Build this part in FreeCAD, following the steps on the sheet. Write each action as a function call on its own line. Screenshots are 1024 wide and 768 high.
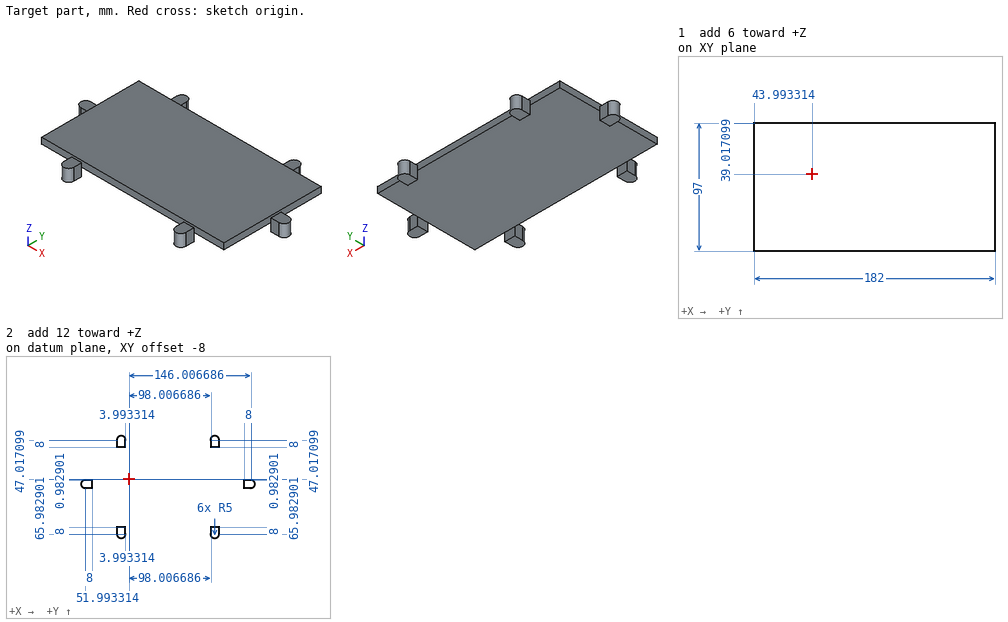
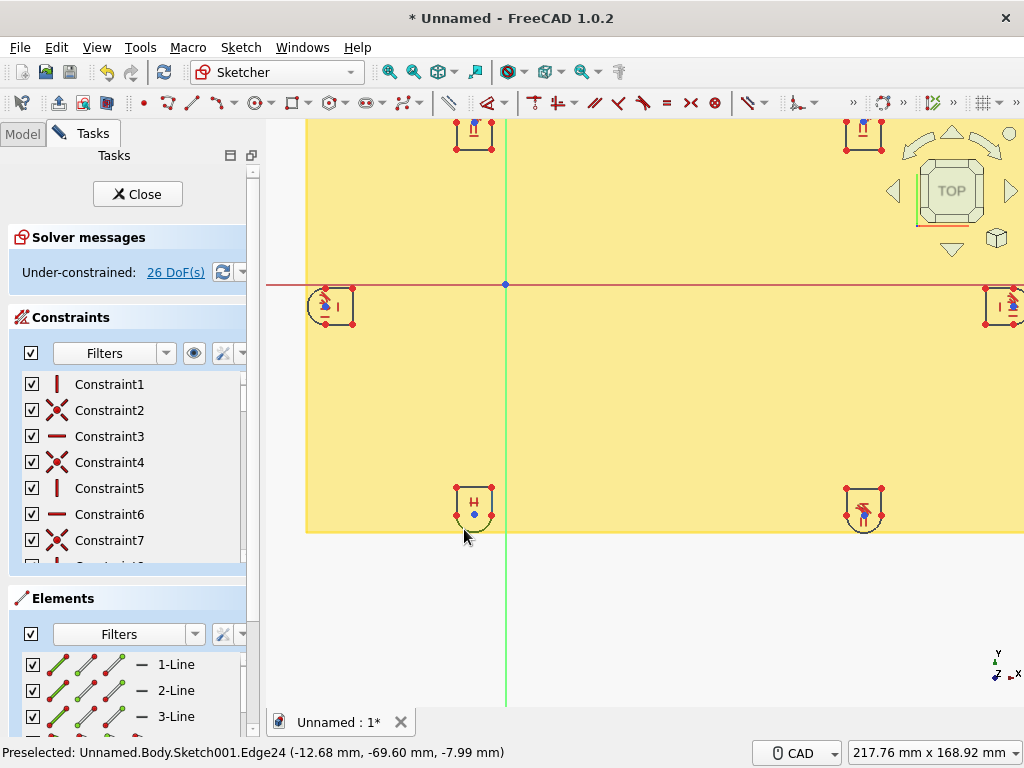
click(644, 104)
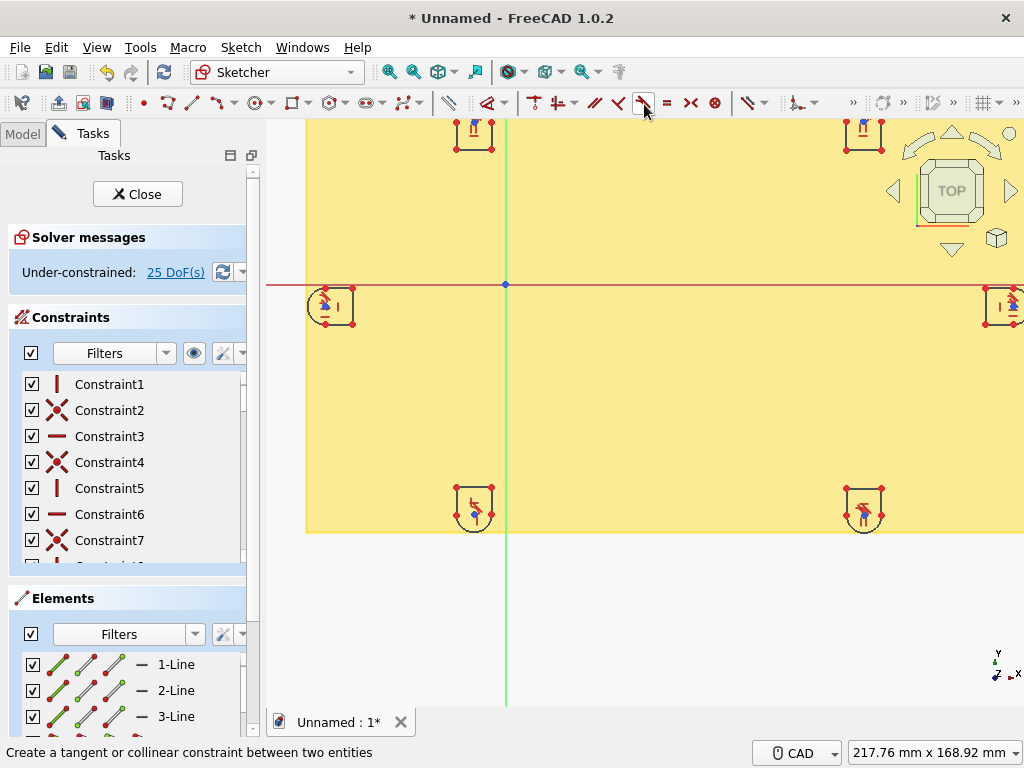
scroll(457, 498, up, 2)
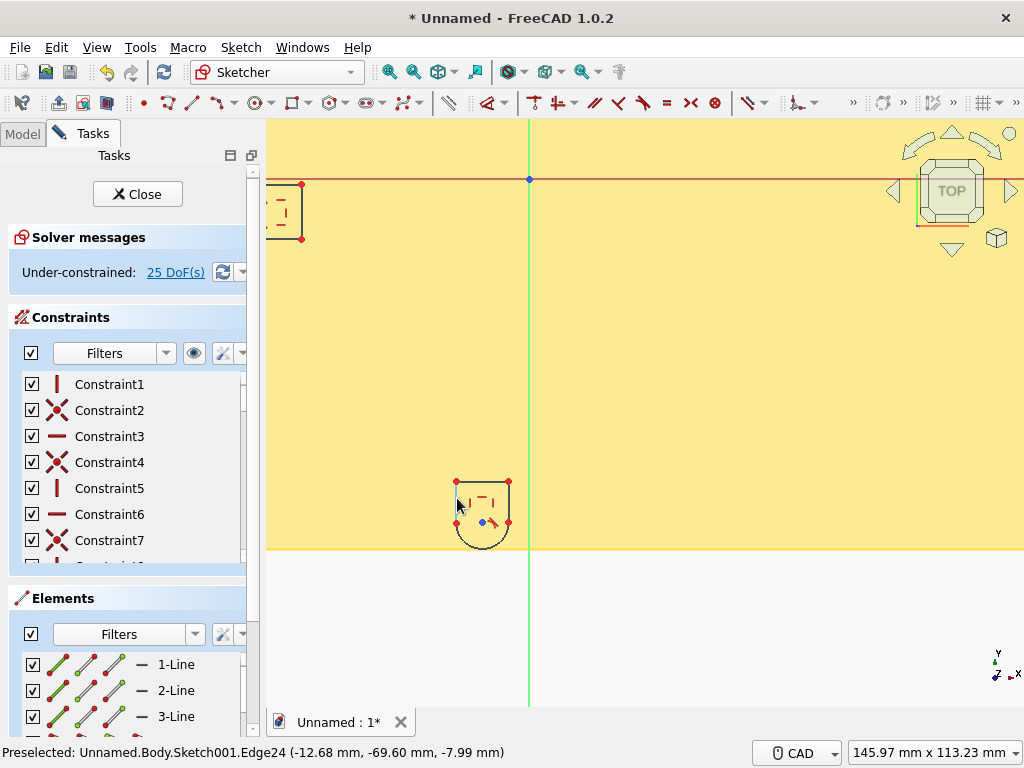
click(456, 498)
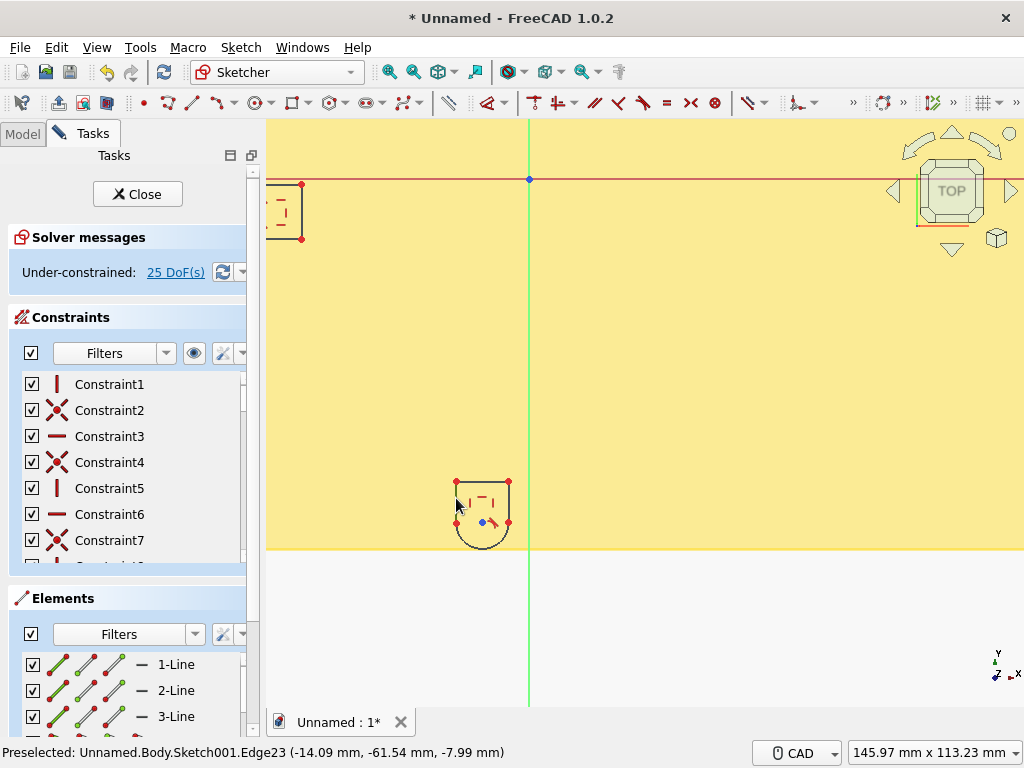
click(467, 544)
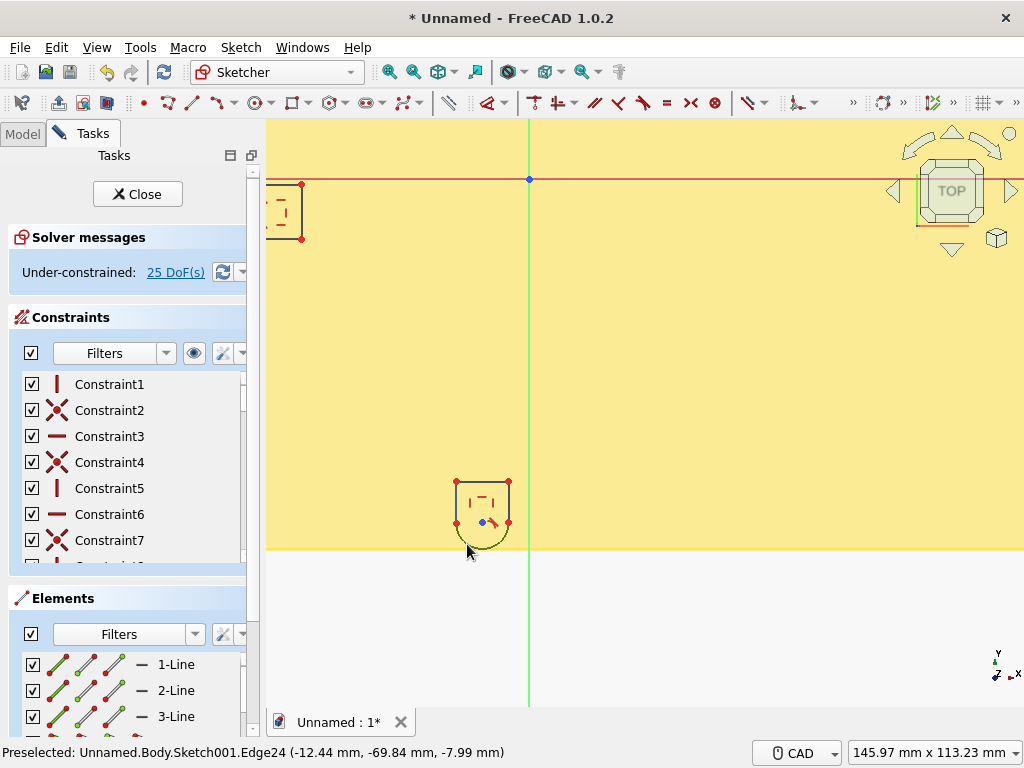
click(644, 104)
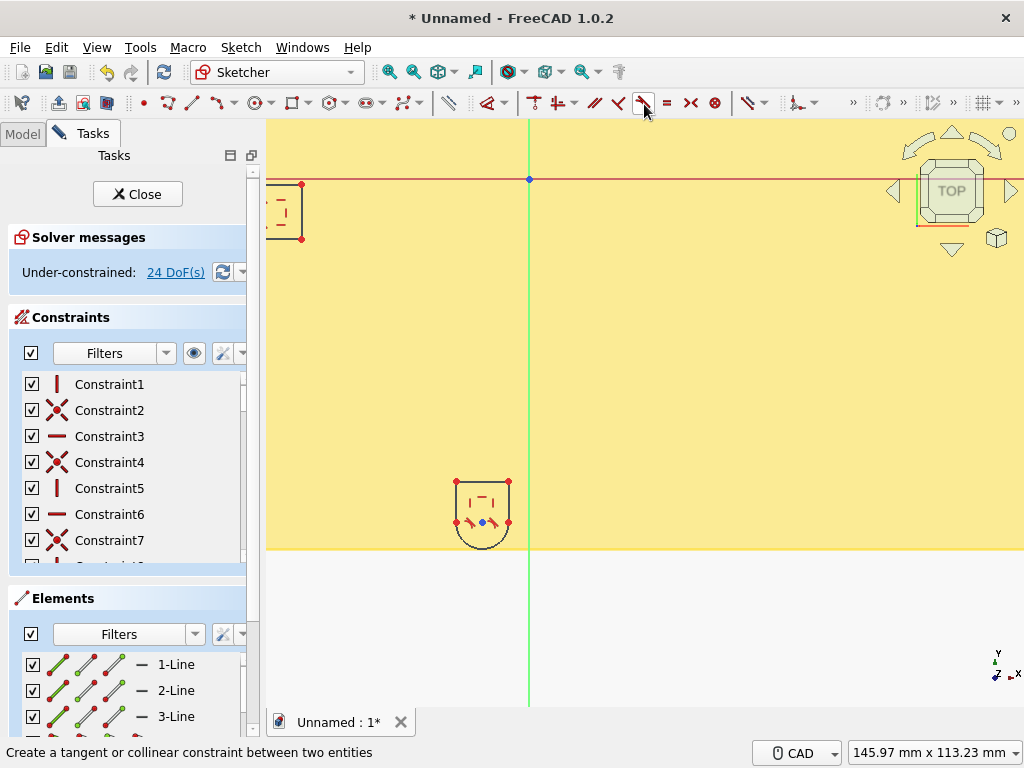
scroll(462, 520, down, 5)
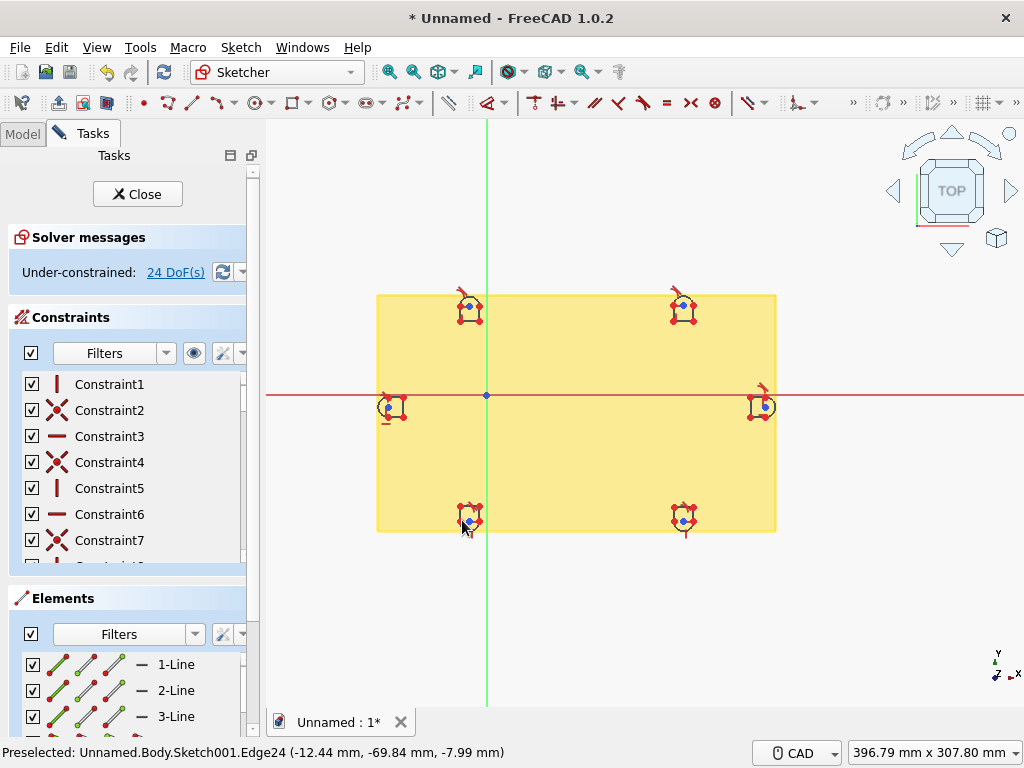
scroll(678, 530, up, 3)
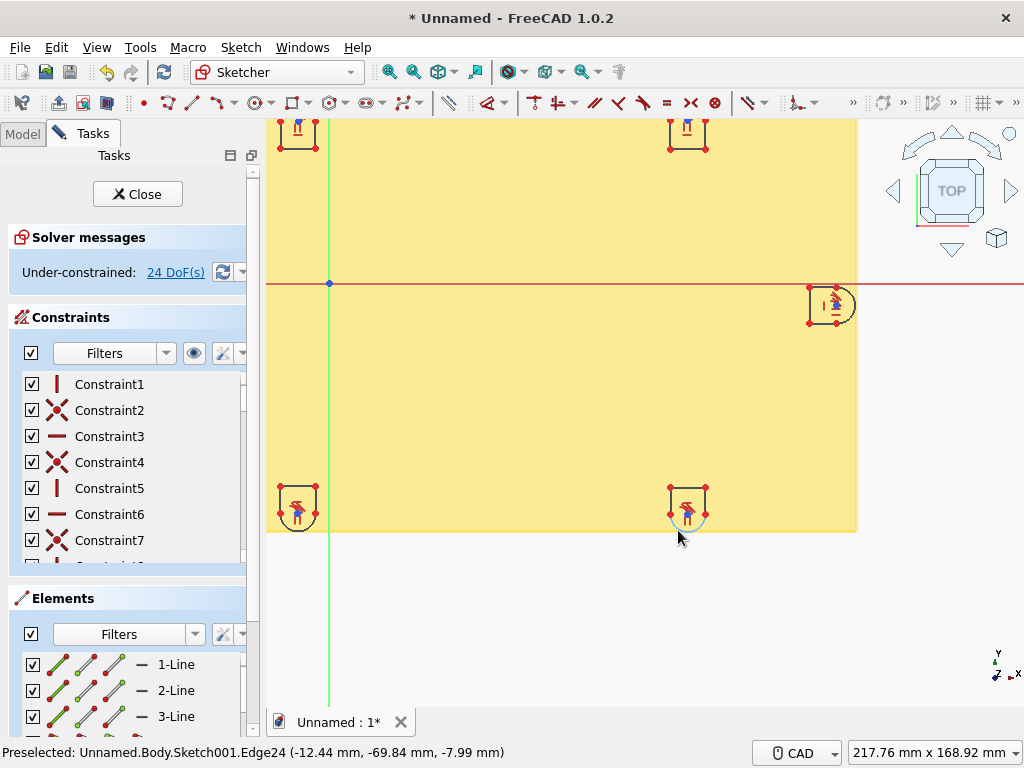
click(678, 529)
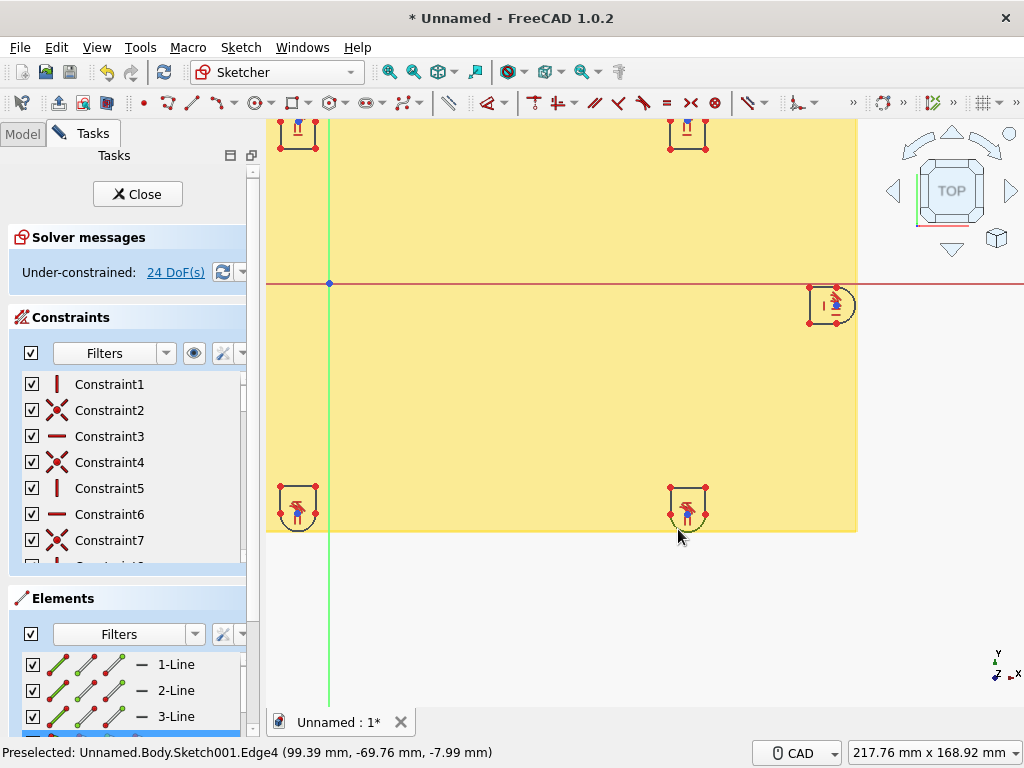
click(852, 316)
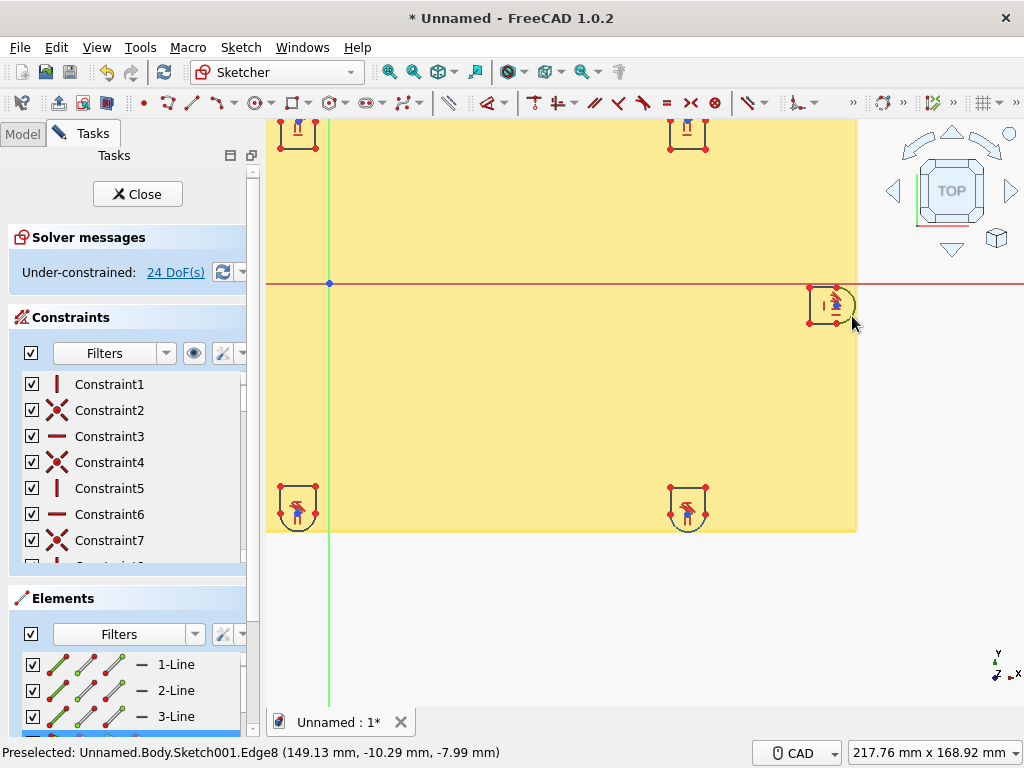
scroll(678, 530, down, 3)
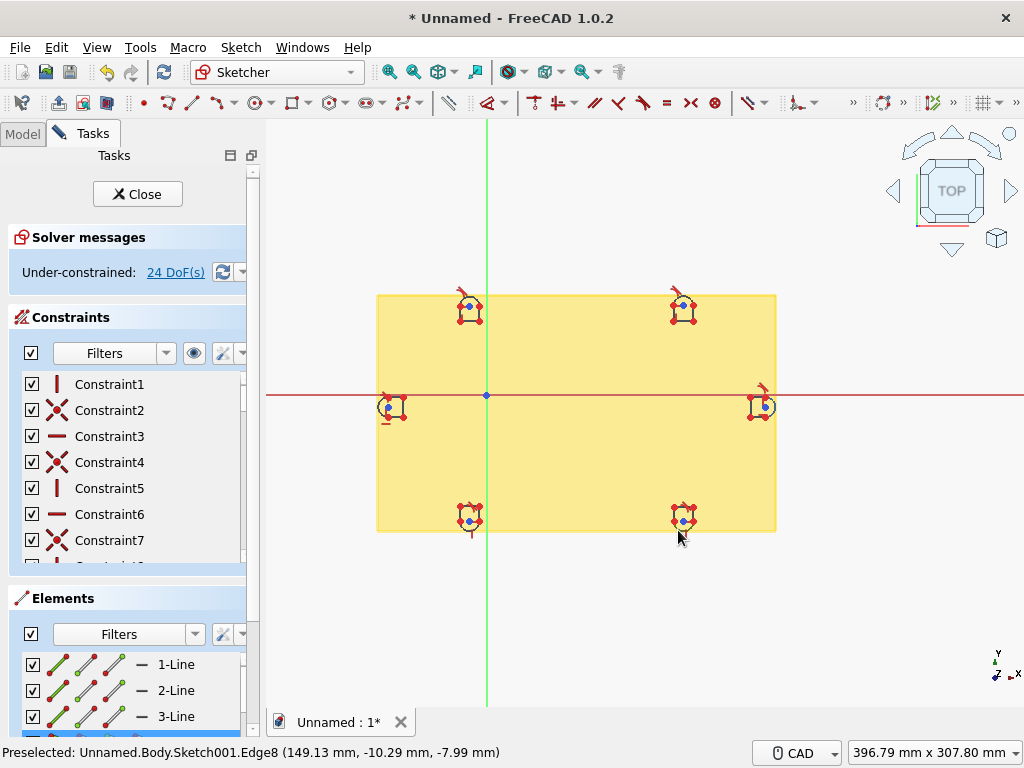
scroll(689, 298, up, 3)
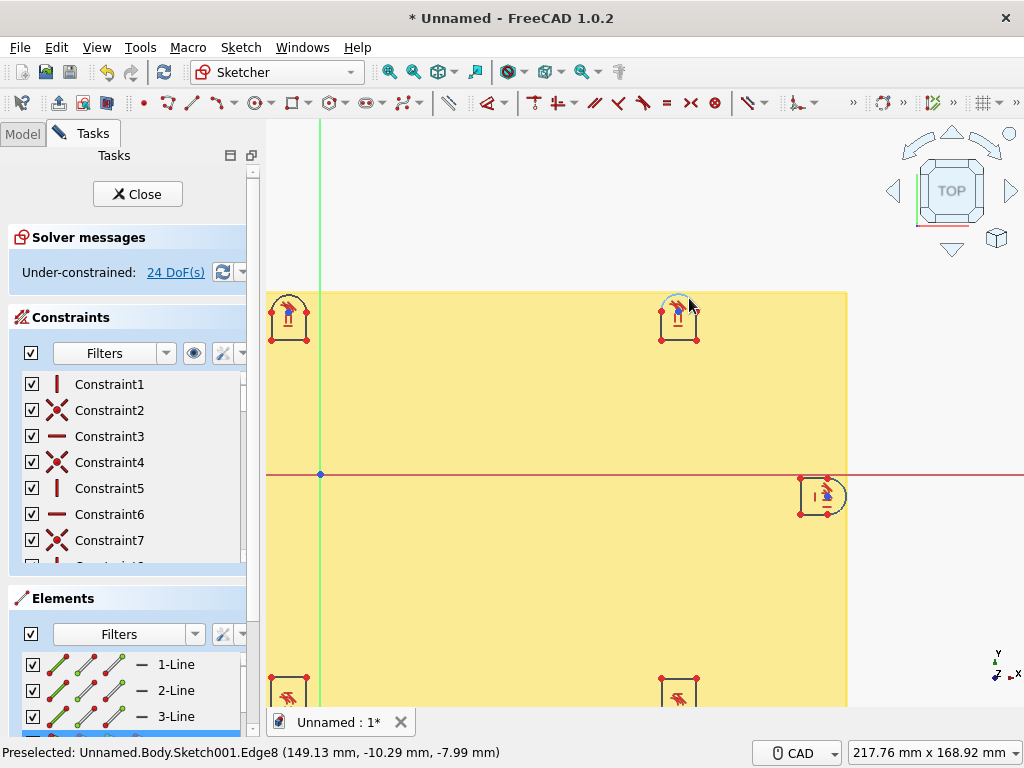
click(689, 298)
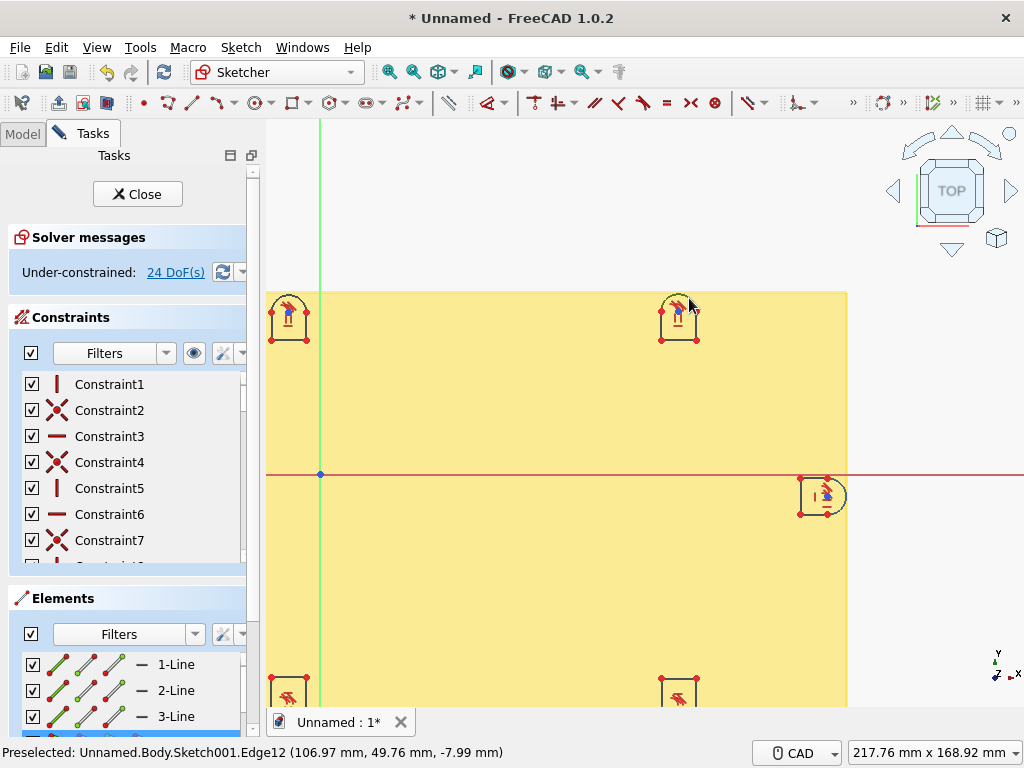
click(299, 299)